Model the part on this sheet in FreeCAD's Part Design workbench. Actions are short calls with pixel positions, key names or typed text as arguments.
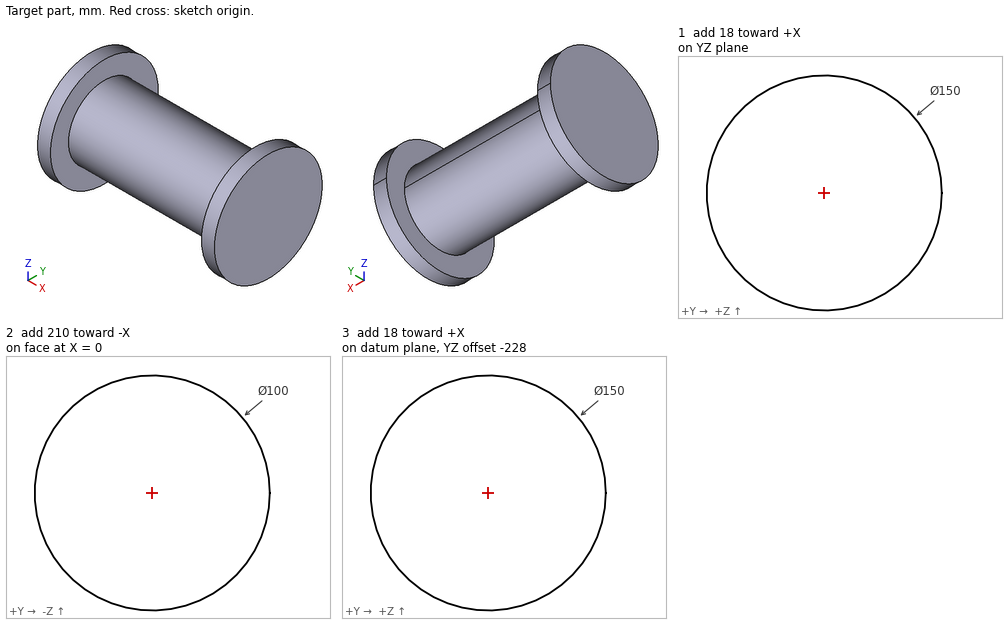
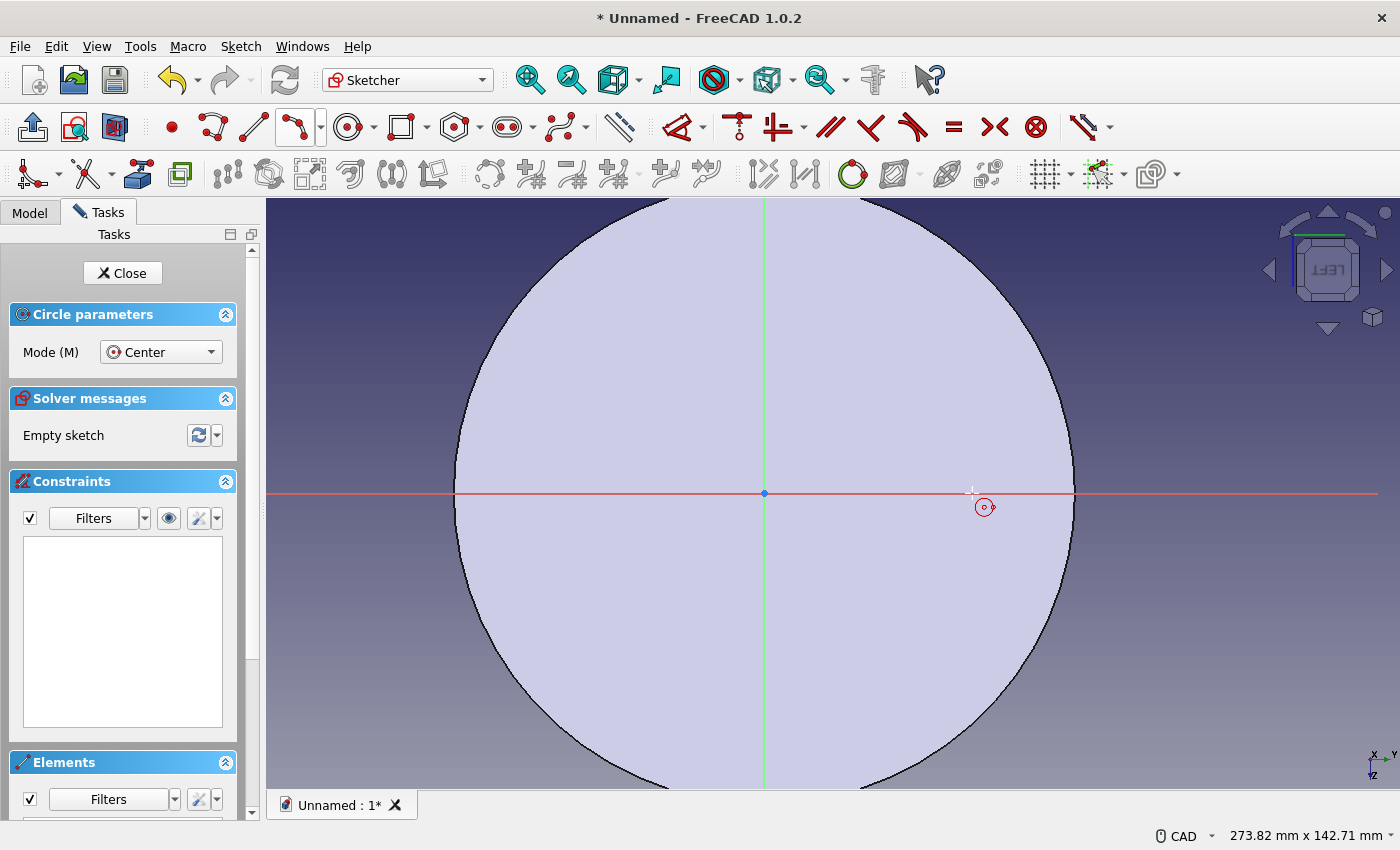
click(764, 494)
move(911, 347)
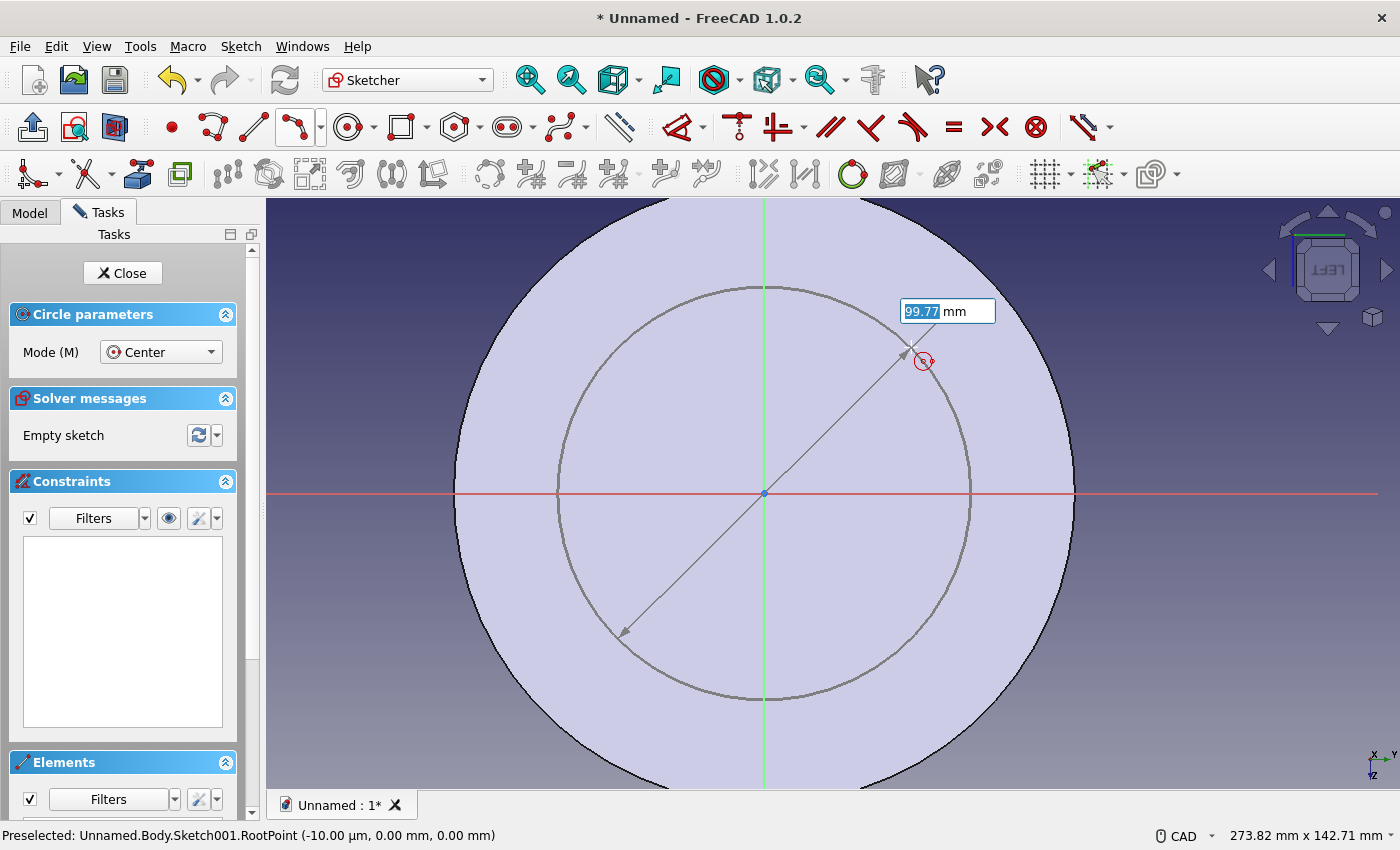
text(100)
key(Return)
key(Escape)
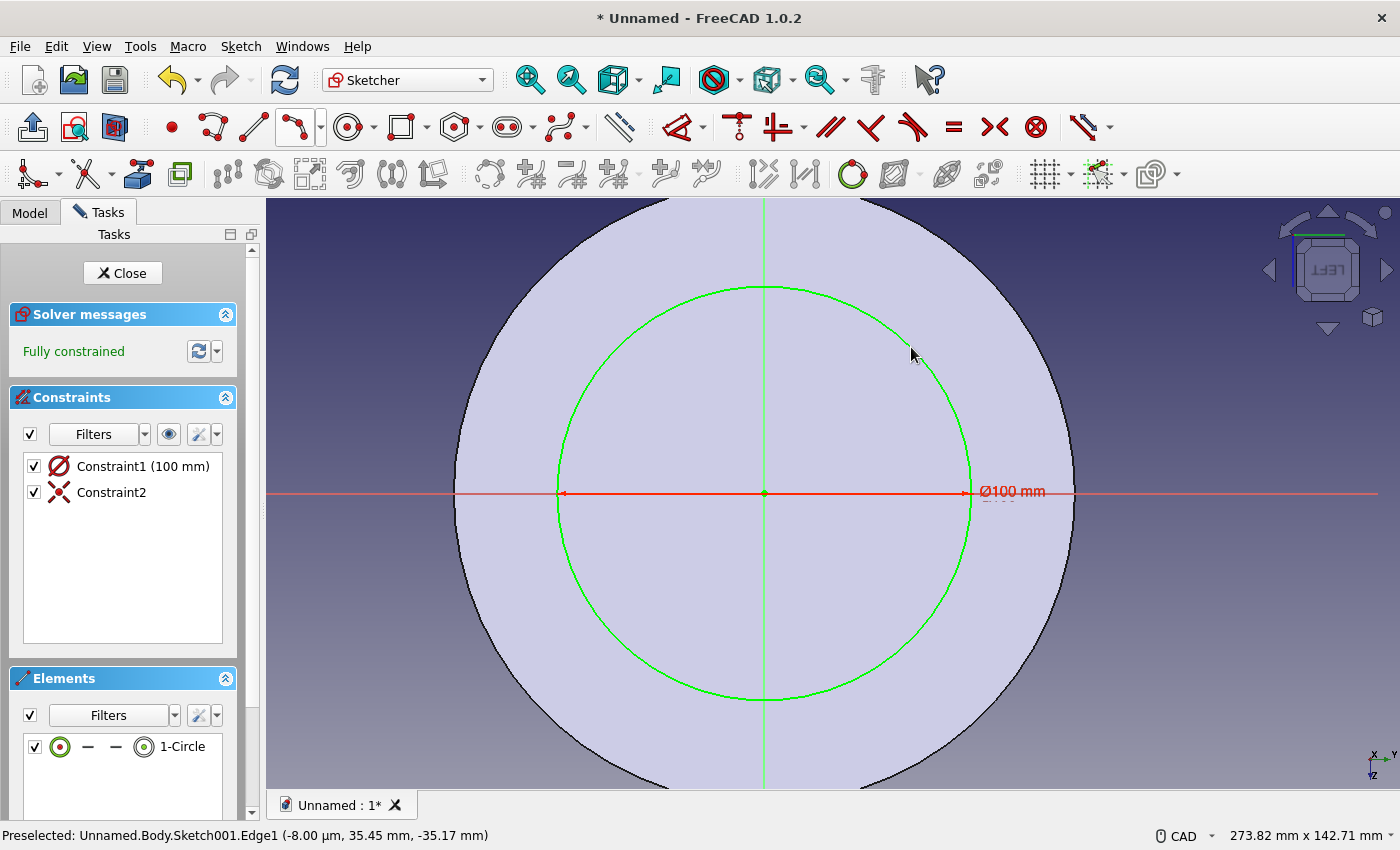
click(123, 273)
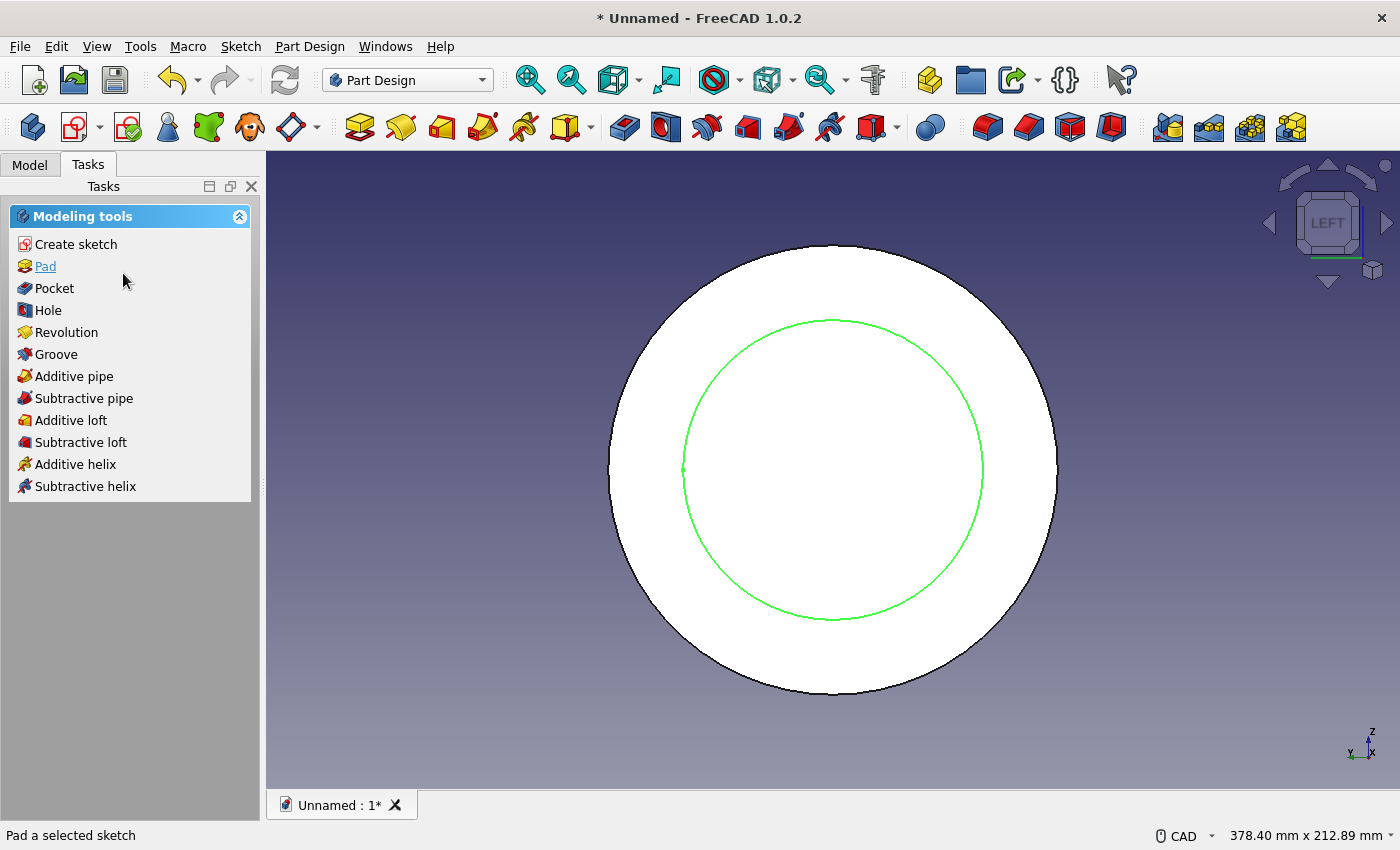
click(360, 128)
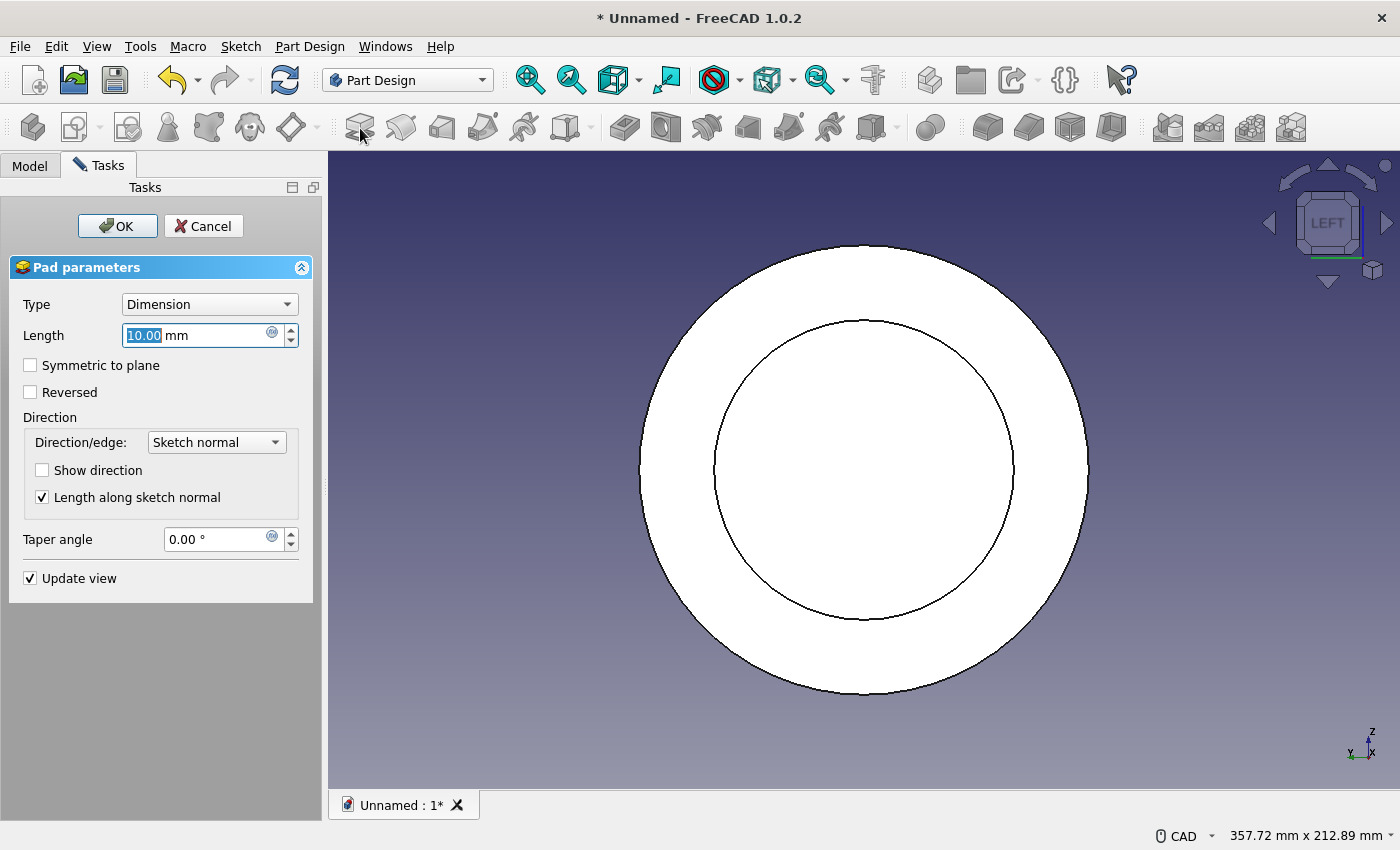
text(210)
key(Tab)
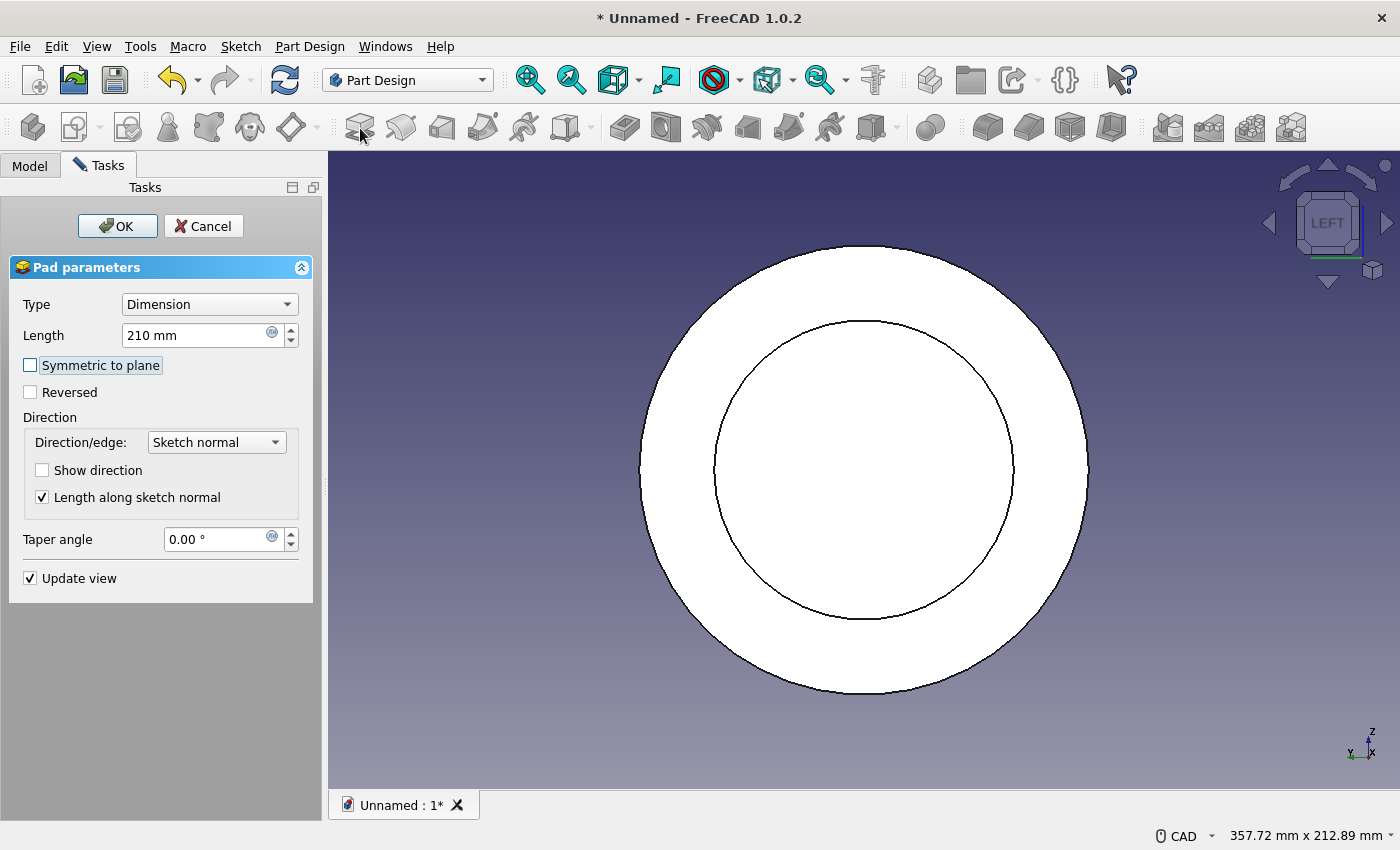
click(118, 226)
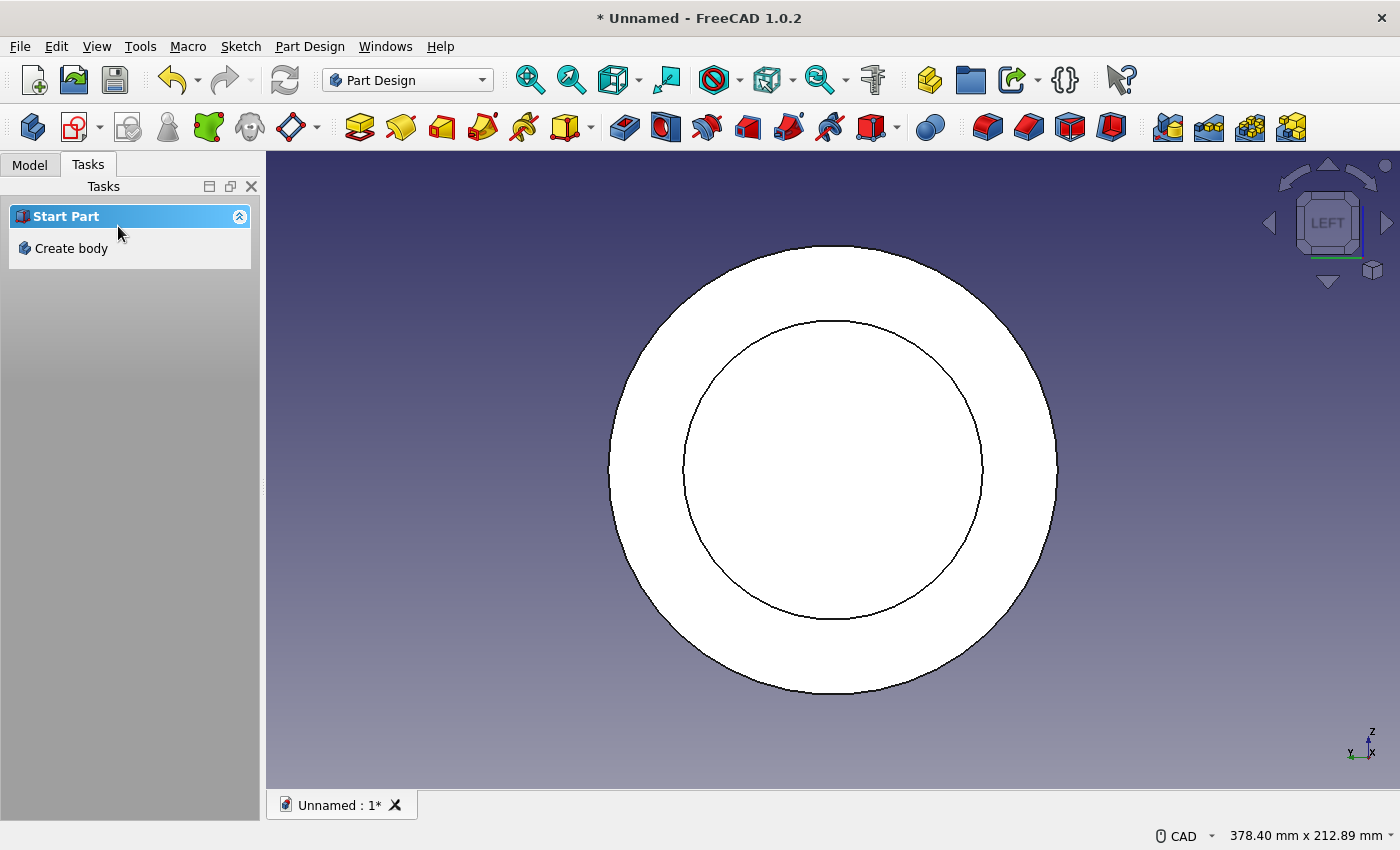
click(30, 164)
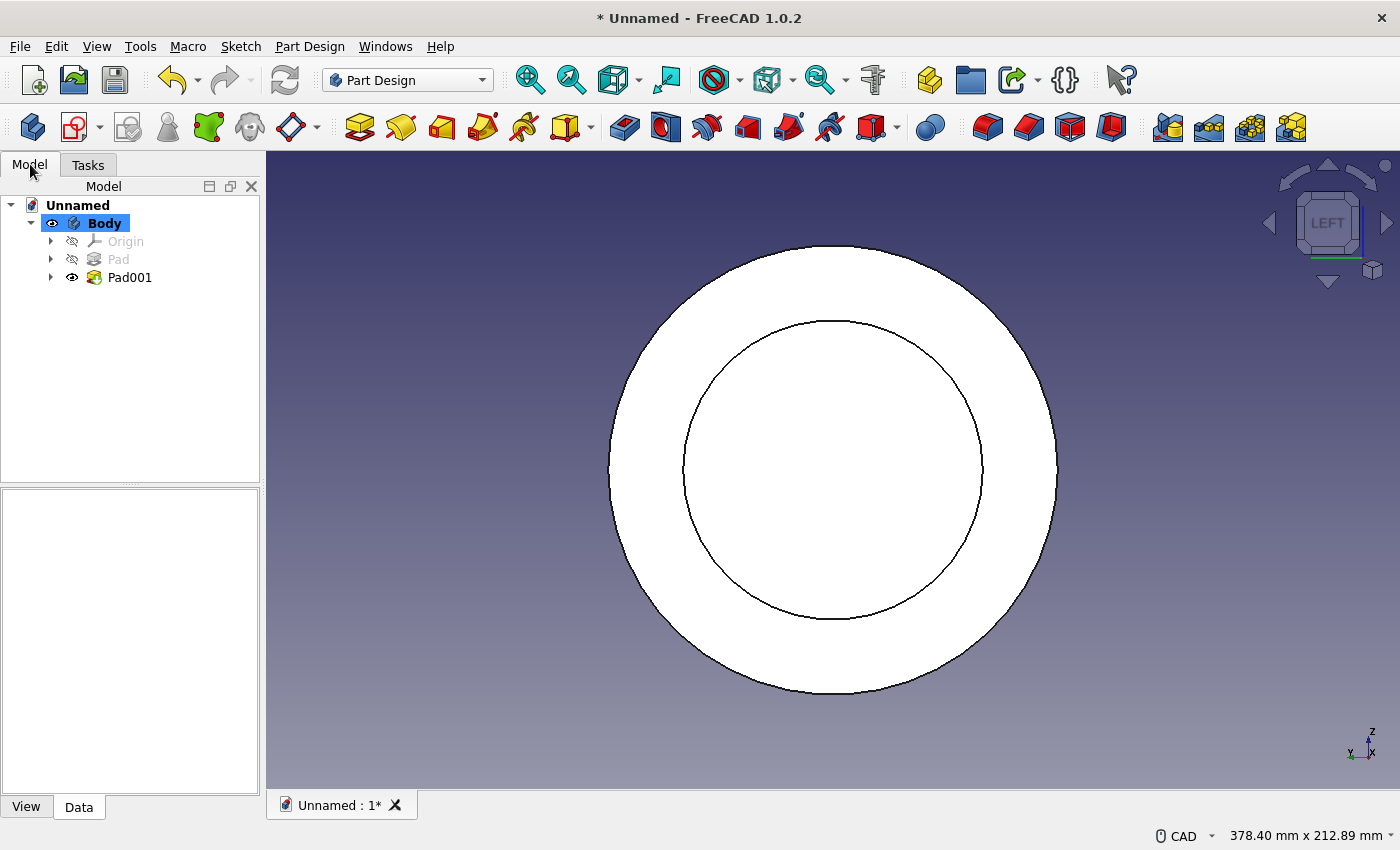
click(51, 241)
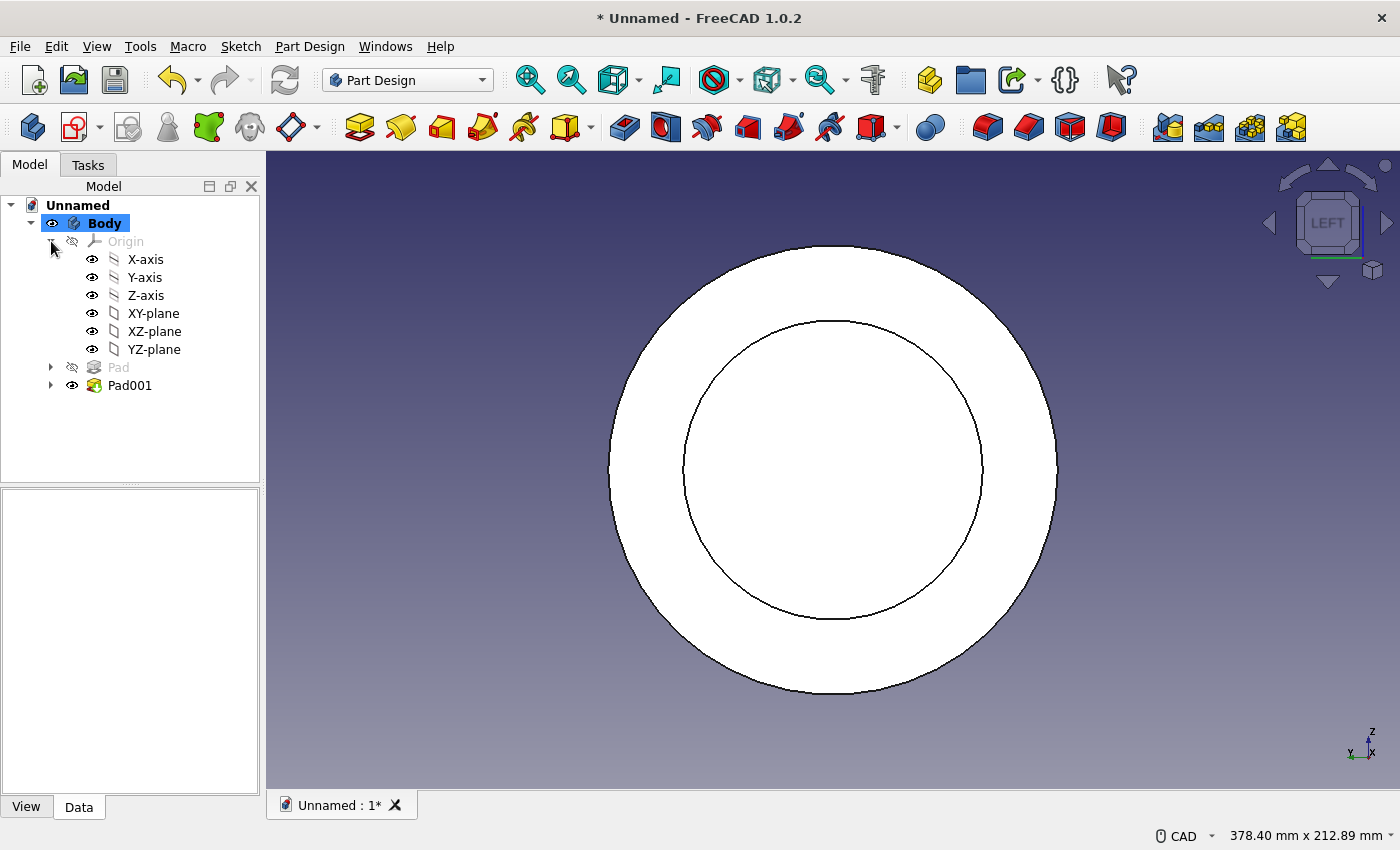
click(137, 349)